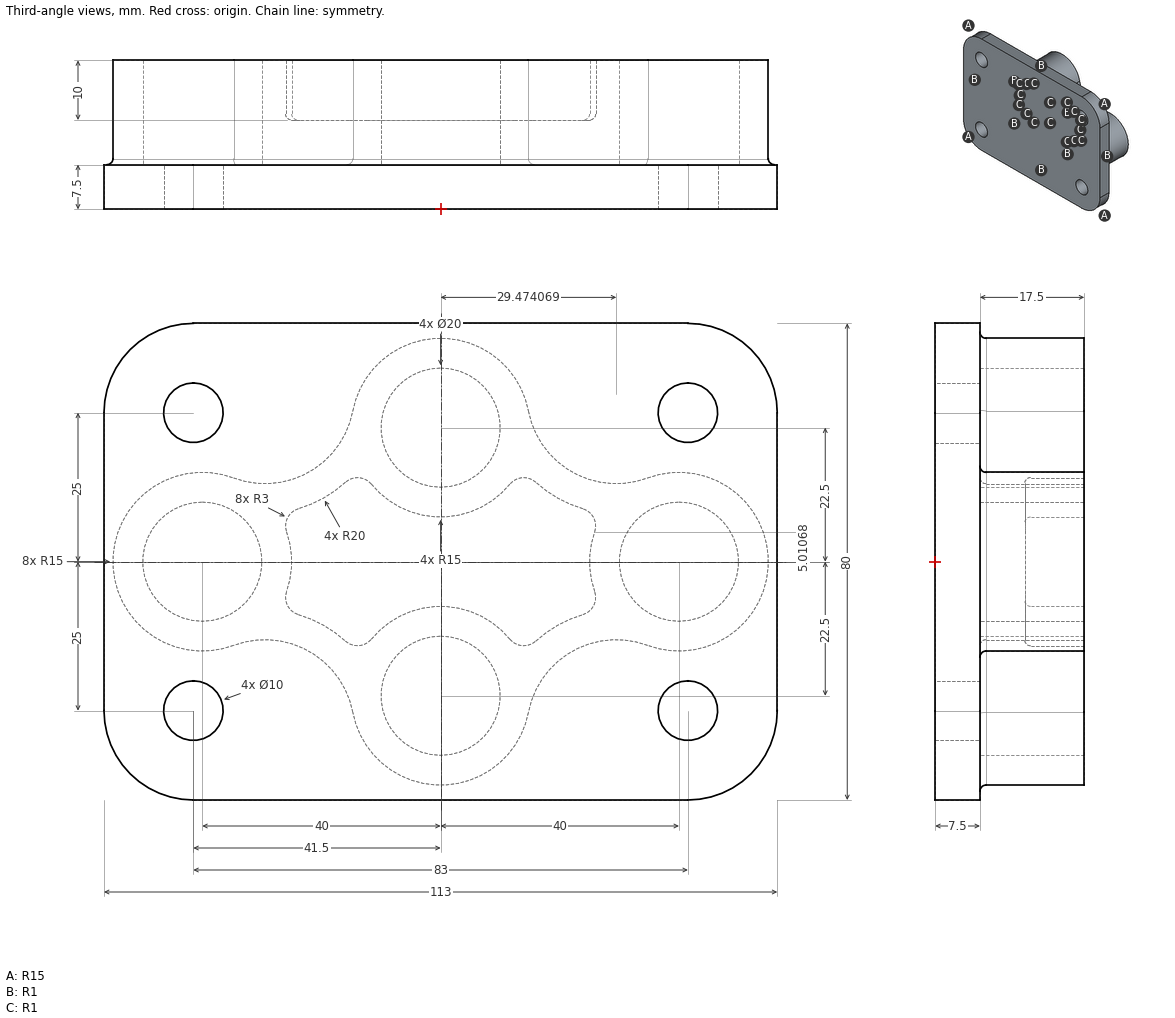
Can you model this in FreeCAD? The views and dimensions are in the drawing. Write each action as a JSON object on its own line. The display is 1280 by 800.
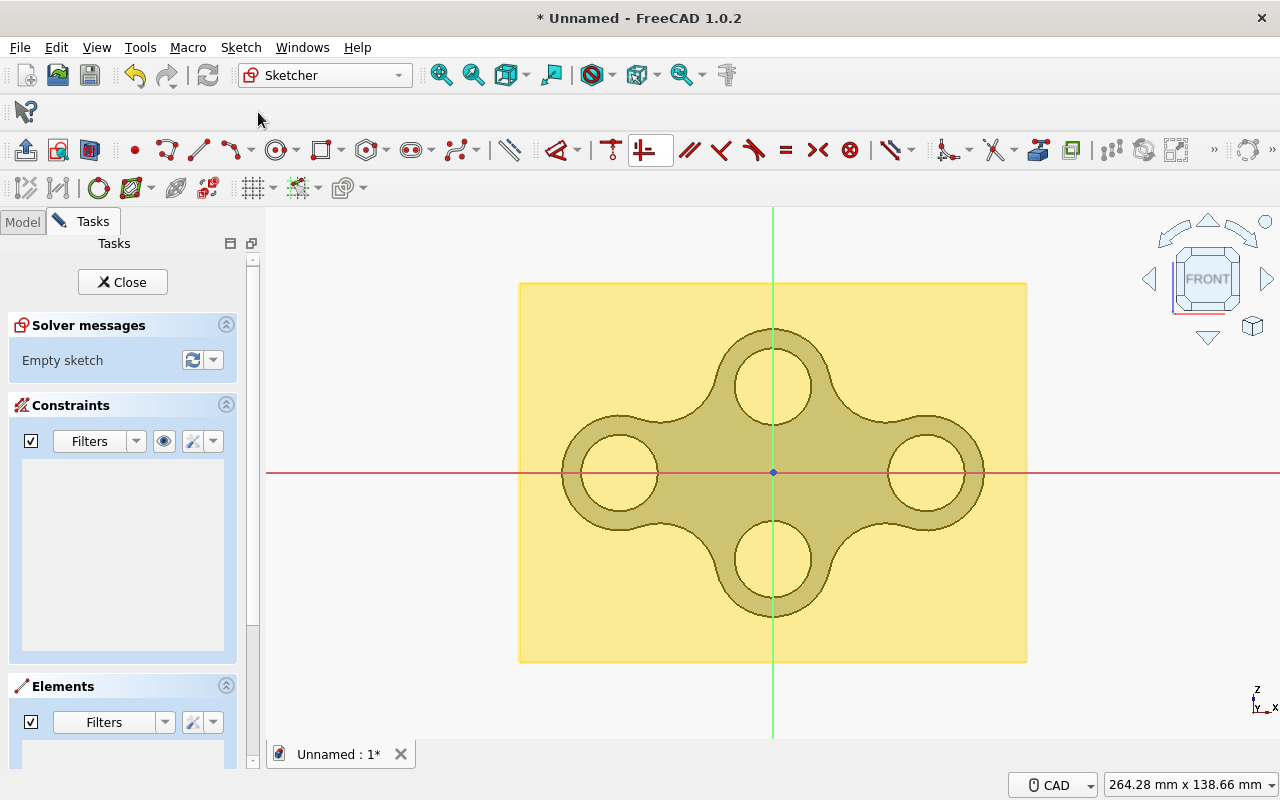
{"action": "scroll", "coordinate": [813, 473], "scroll_direction": "up", "scroll_amount": 5}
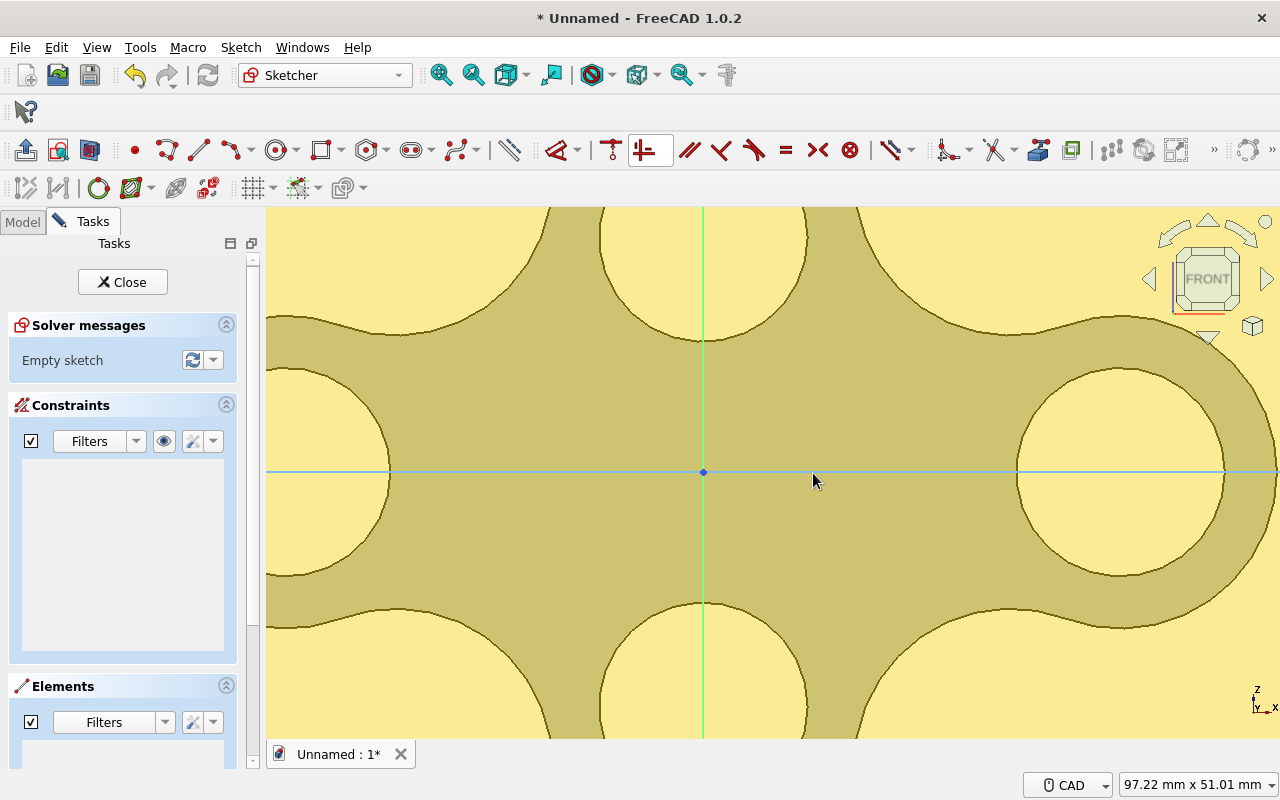
{"action": "key", "text": "g 3 a"}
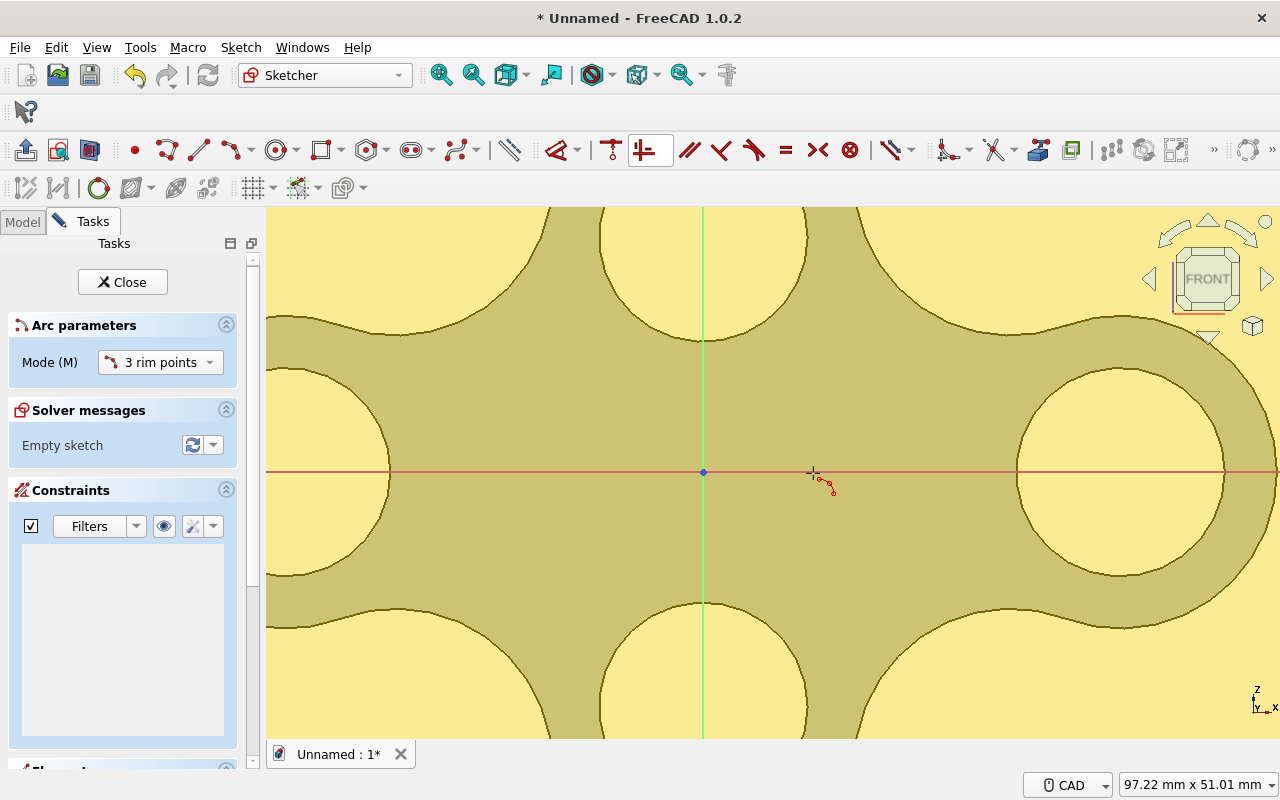
{"action": "left_click", "coordinate": [582, 336]}
{"action": "left_click", "coordinate": [825, 336]}
{"action": "left_click", "coordinate": [676, 391]}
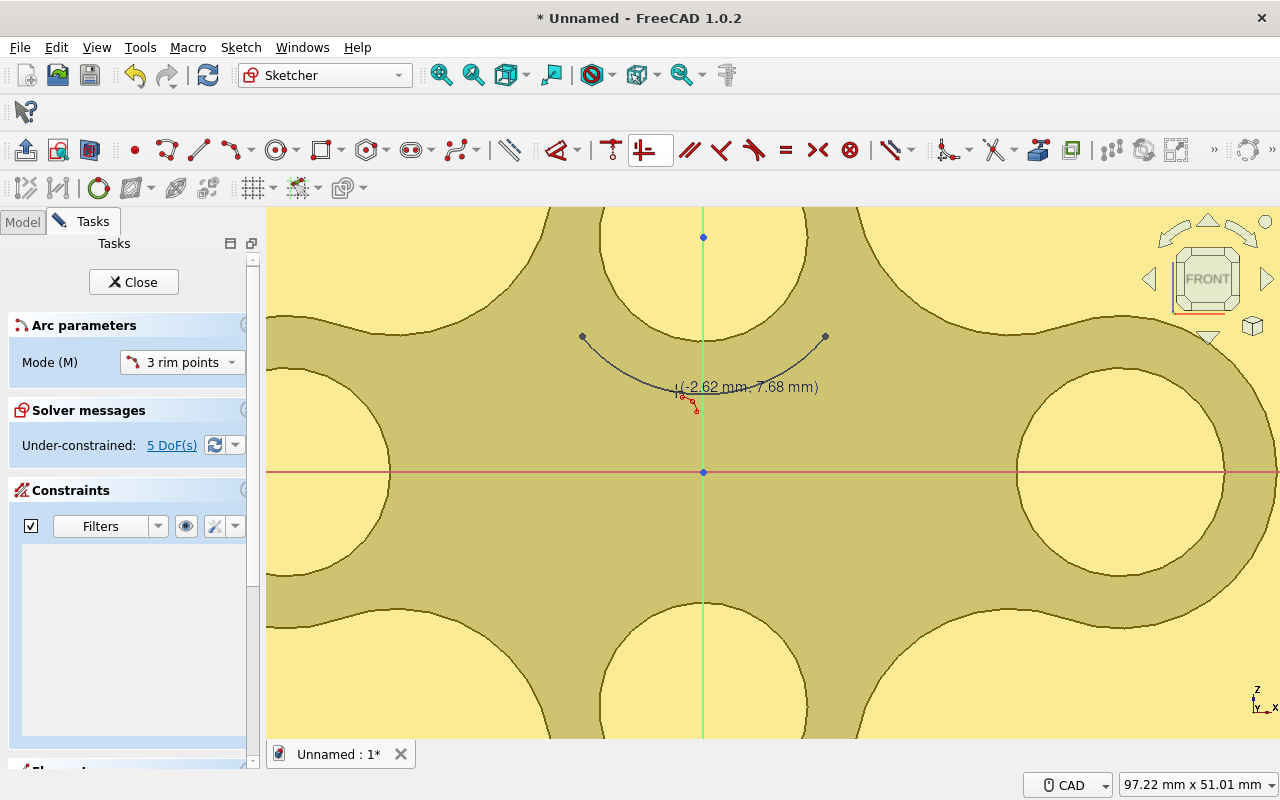
{"action": "left_click", "coordinate": [825, 337]}
{"action": "left_click", "coordinate": [870, 333]}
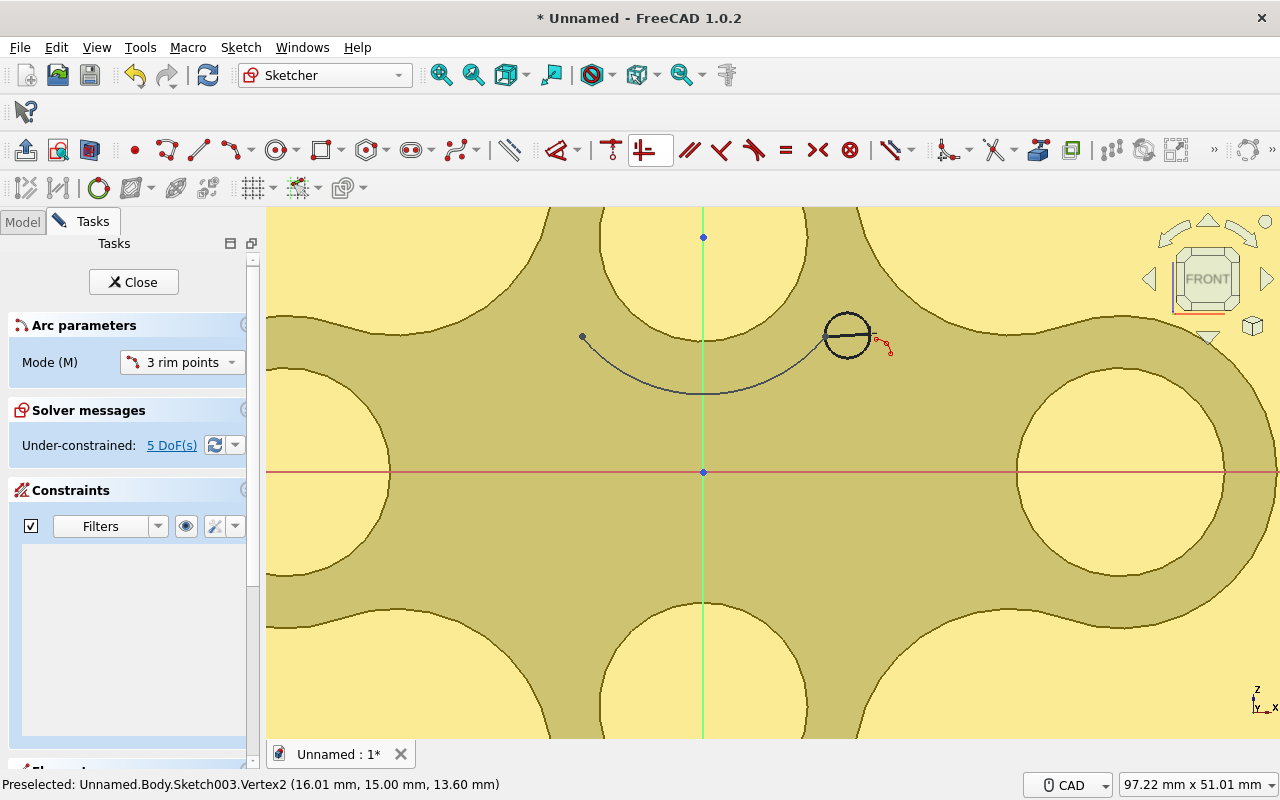
{"action": "scroll", "coordinate": [847, 325], "scroll_direction": "up", "scroll_amount": 3}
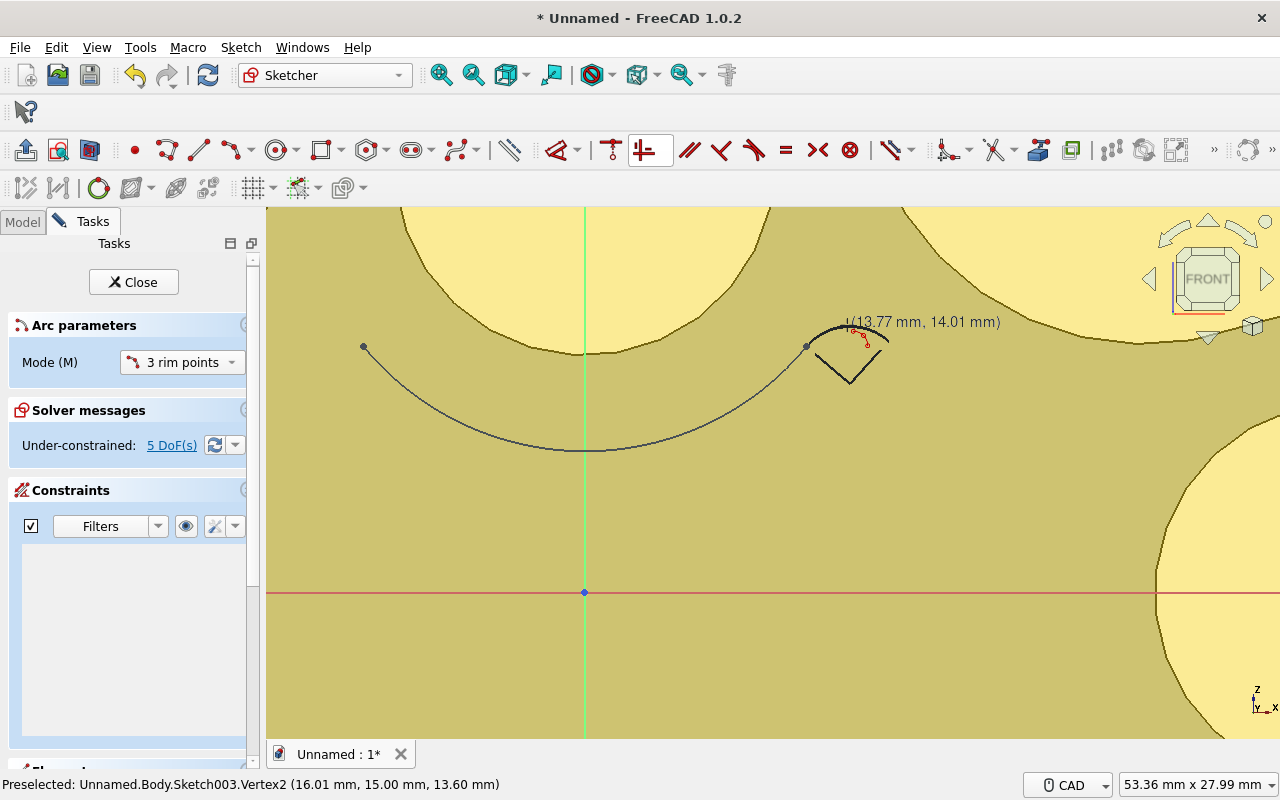
{"action": "left_click", "coordinate": [846, 325]}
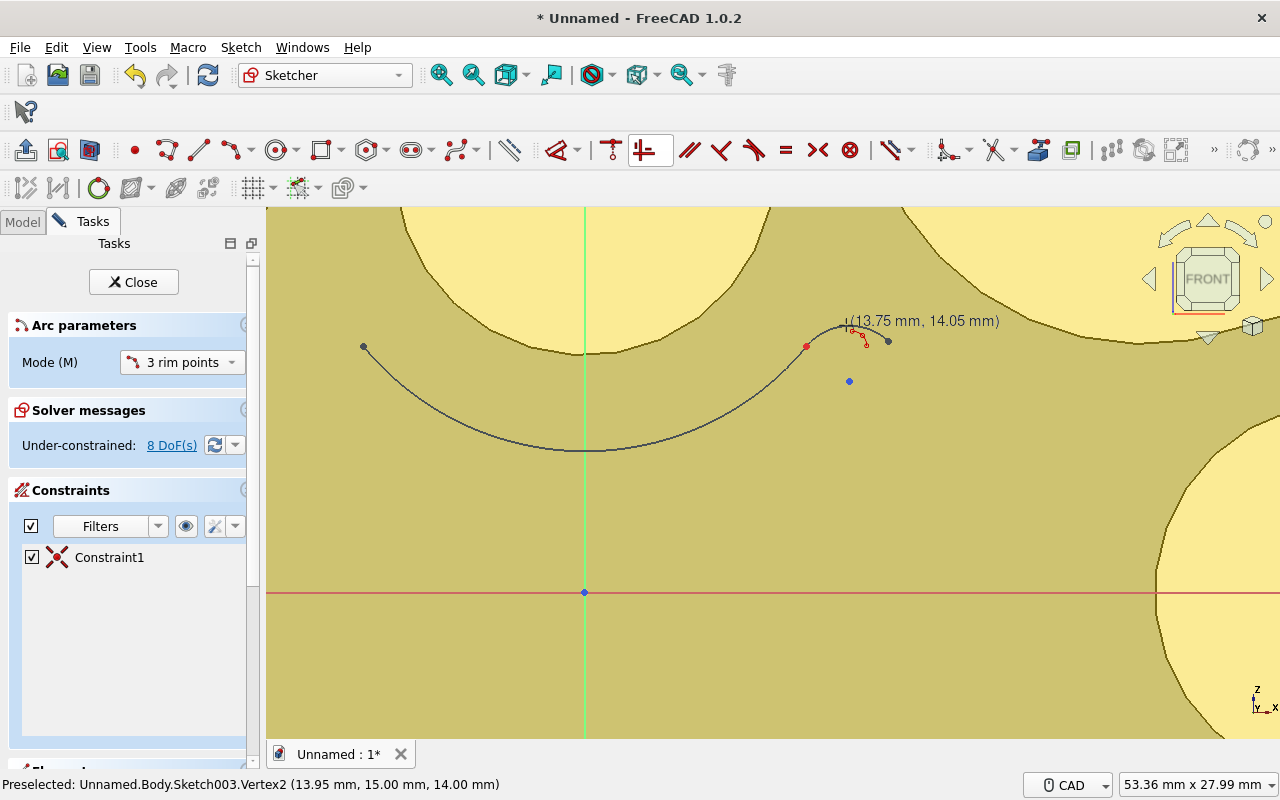
{"action": "left_click", "coordinate": [888, 341]}
{"action": "left_click", "coordinate": [1038, 424]}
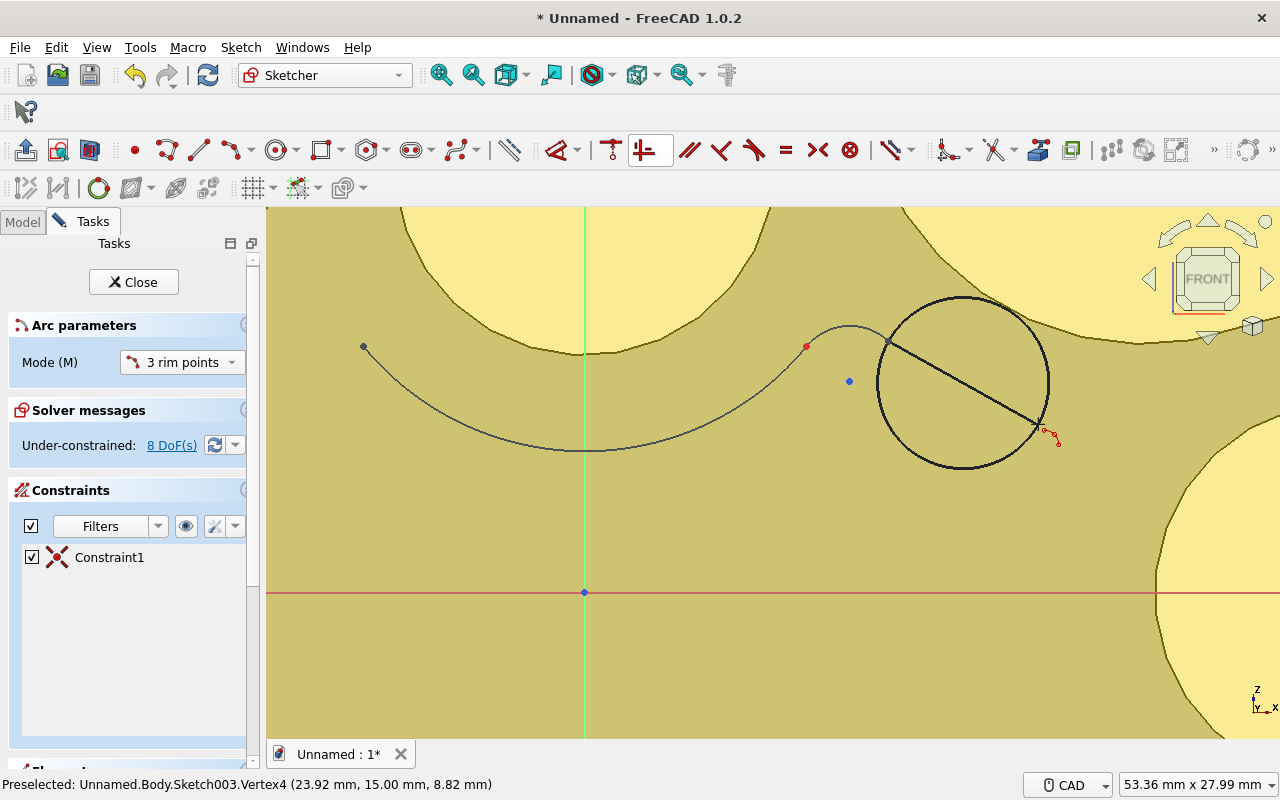
{"action": "scroll", "coordinate": [959, 390], "scroll_direction": "up", "scroll_amount": 3}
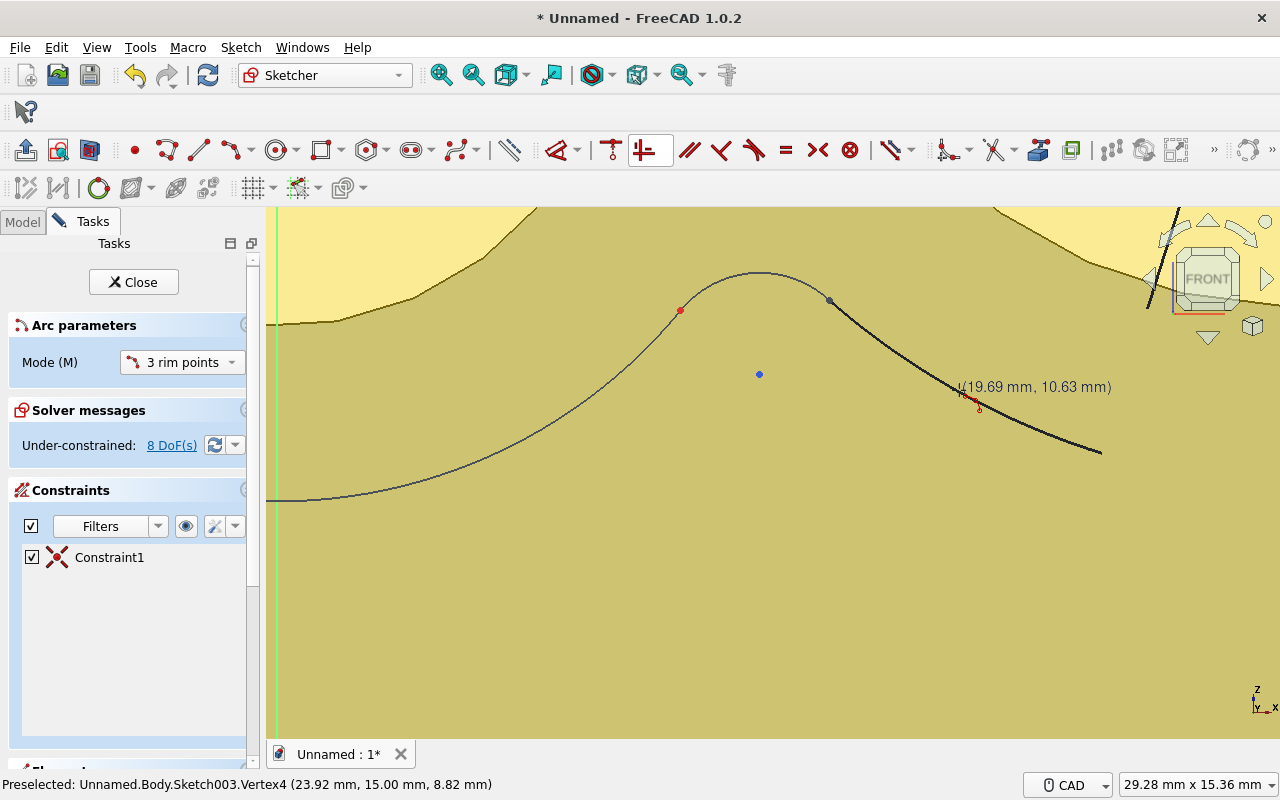
{"action": "left_click", "coordinate": [958, 390]}